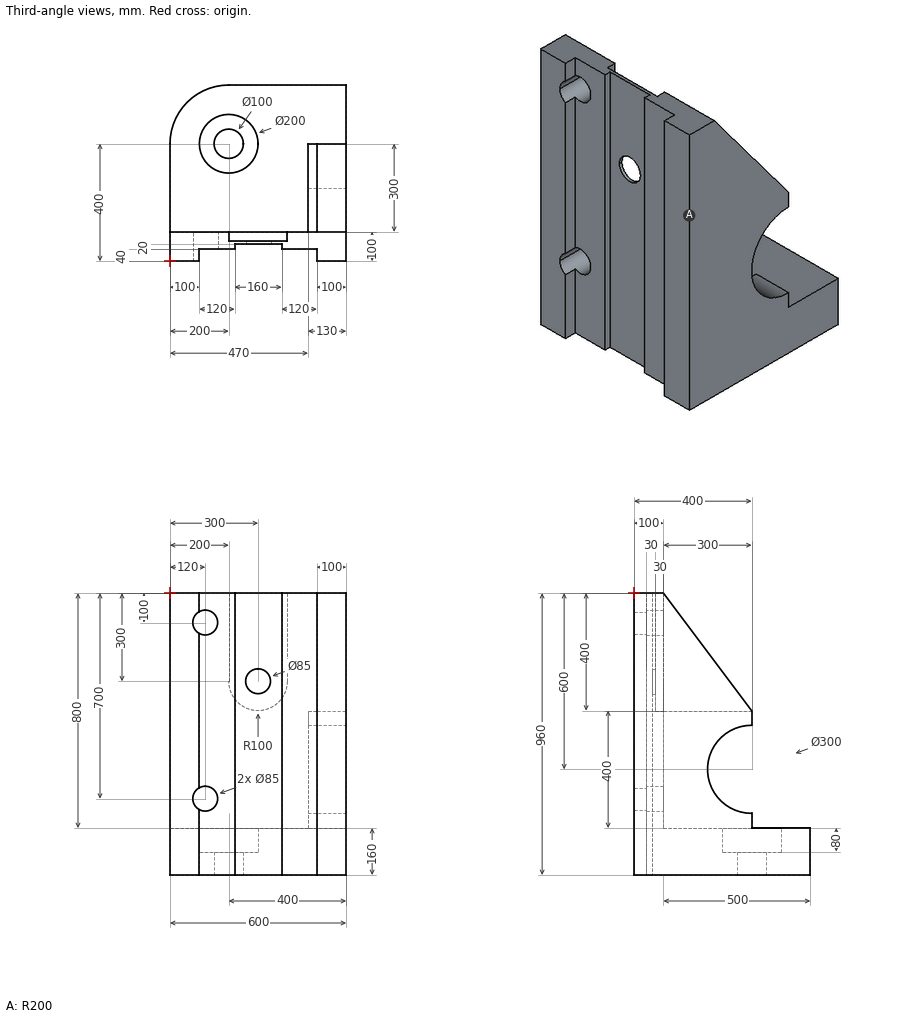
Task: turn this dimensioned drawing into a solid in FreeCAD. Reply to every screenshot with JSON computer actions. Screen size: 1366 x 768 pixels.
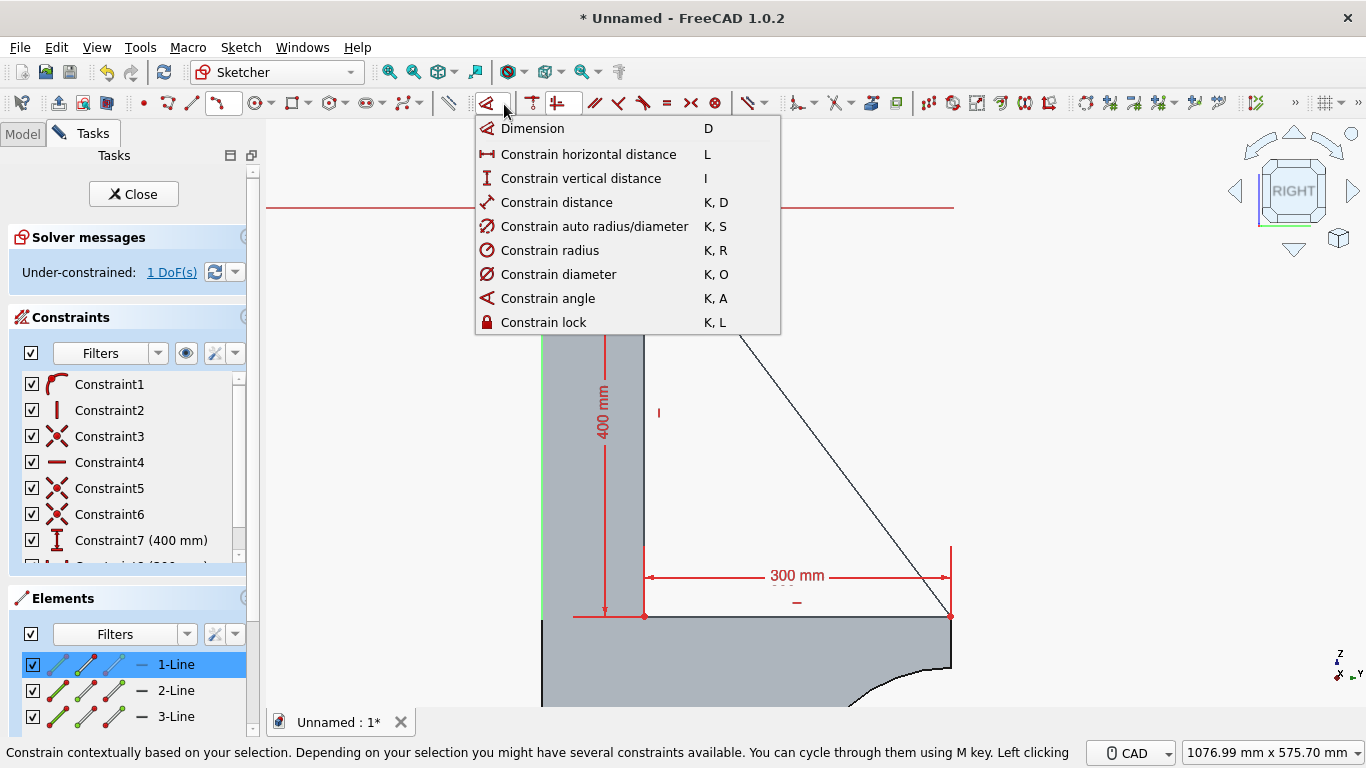
{"action": "left_click", "coordinate": [628, 154]}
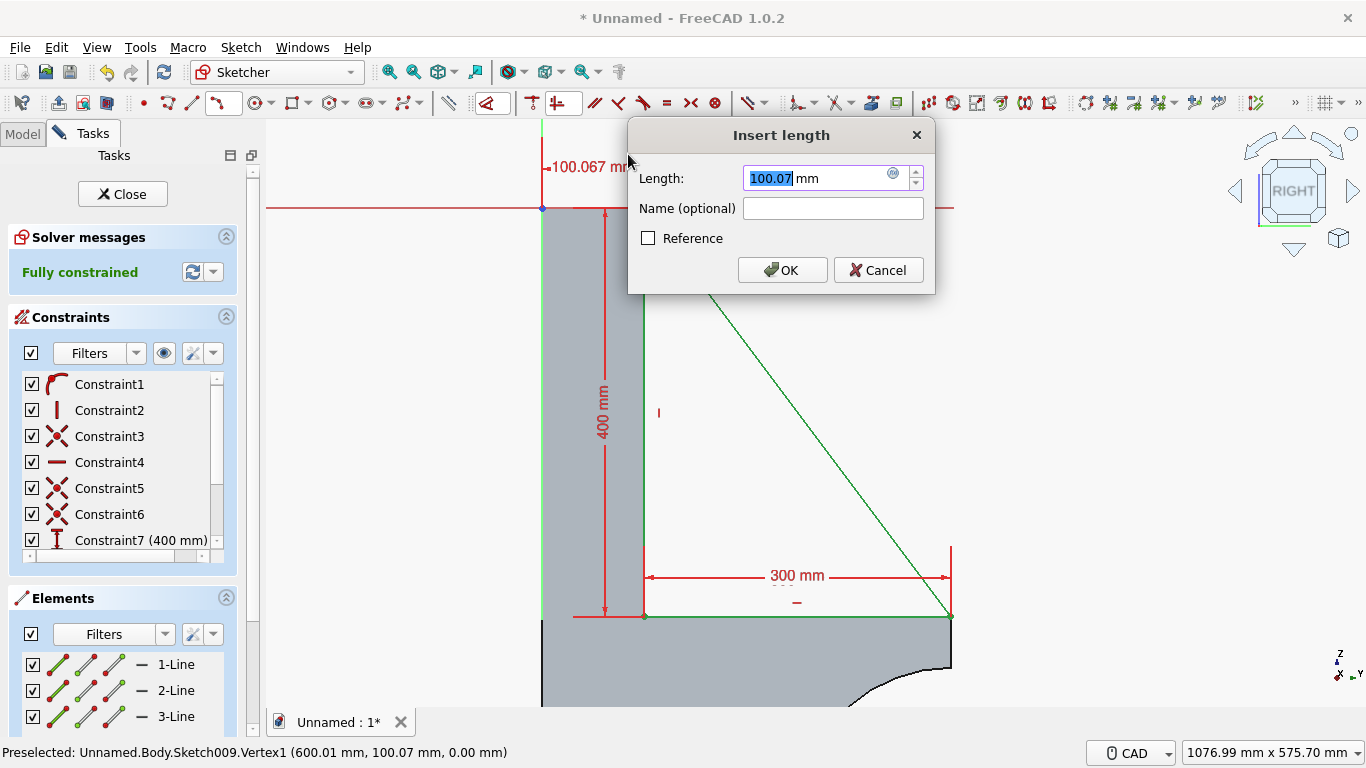
{"action": "type", "text": "100"}
{"action": "key", "text": "Return"}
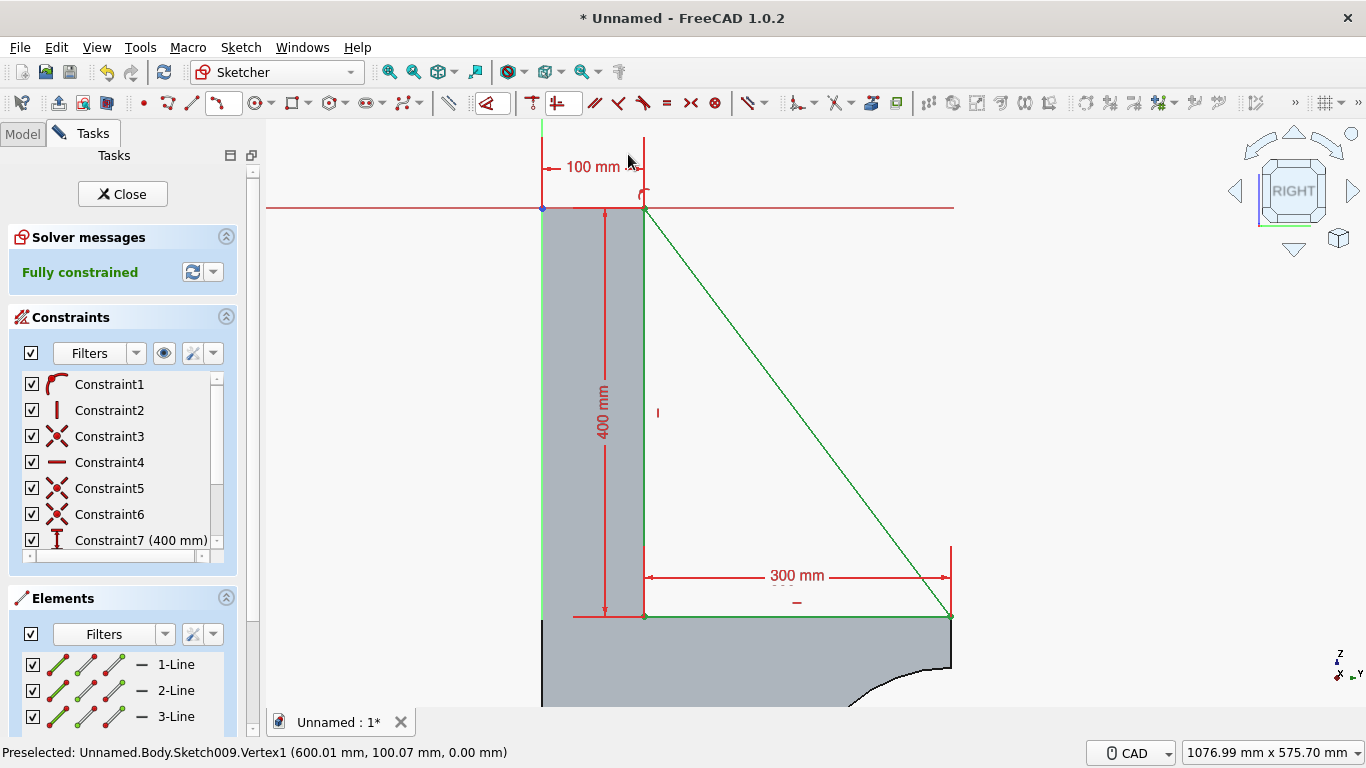
{"action": "left_click", "coordinate": [123, 194]}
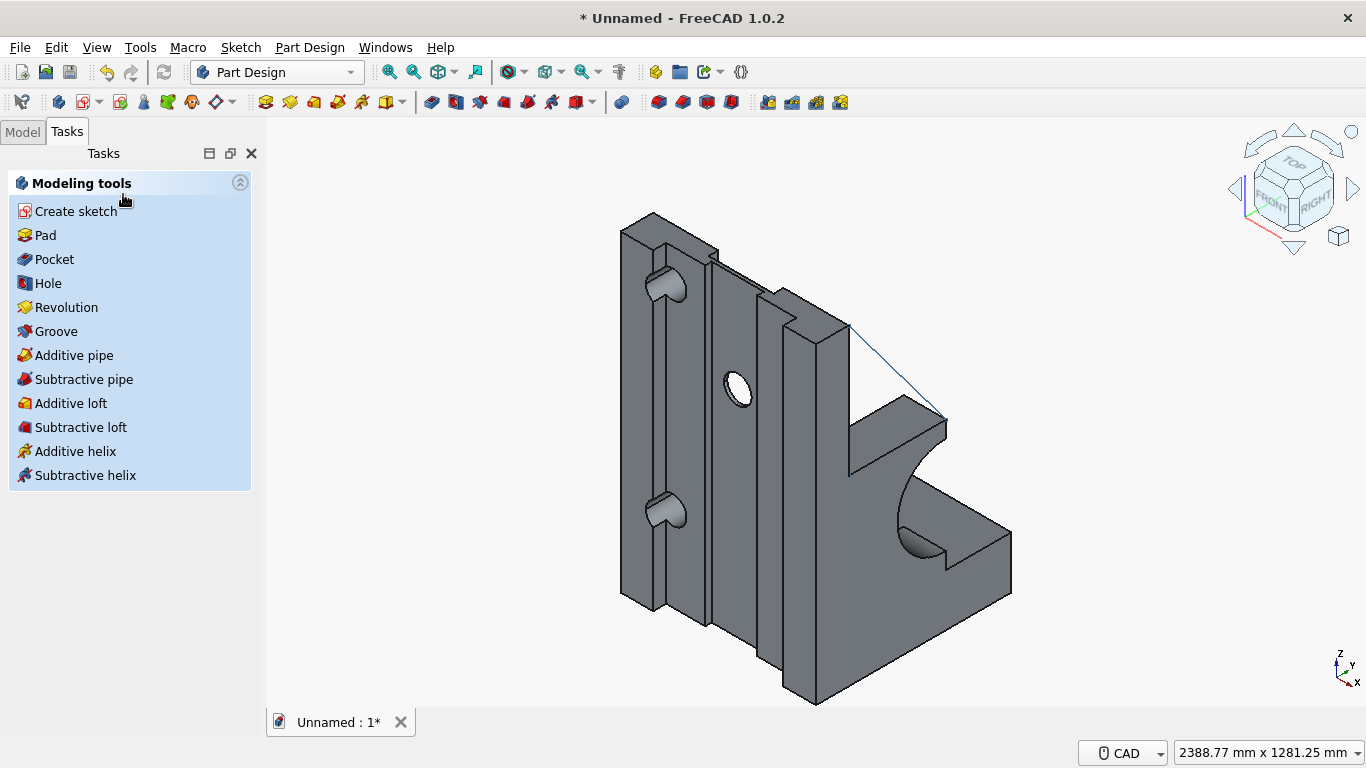
{"action": "left_click", "coordinate": [266, 102]}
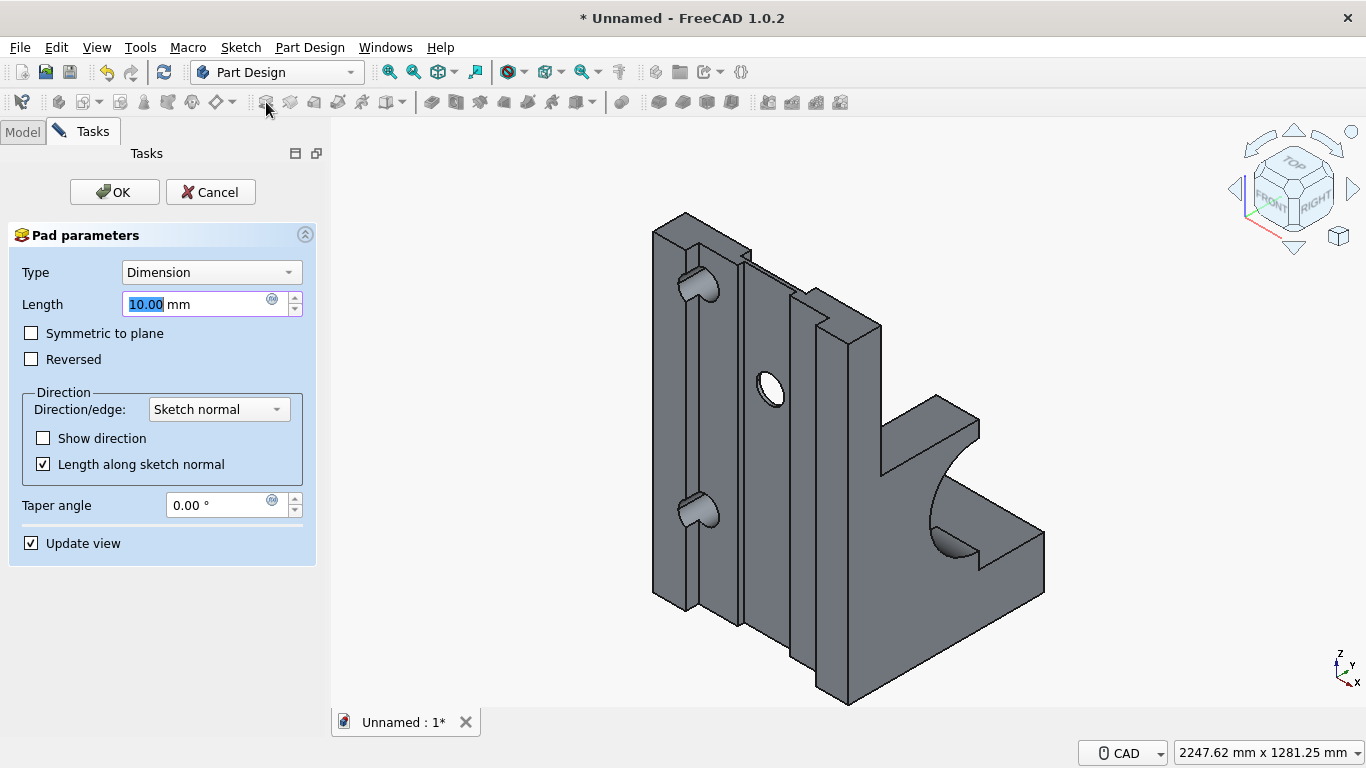
{"action": "type", "text": "100"}
{"action": "key", "text": "Tab"}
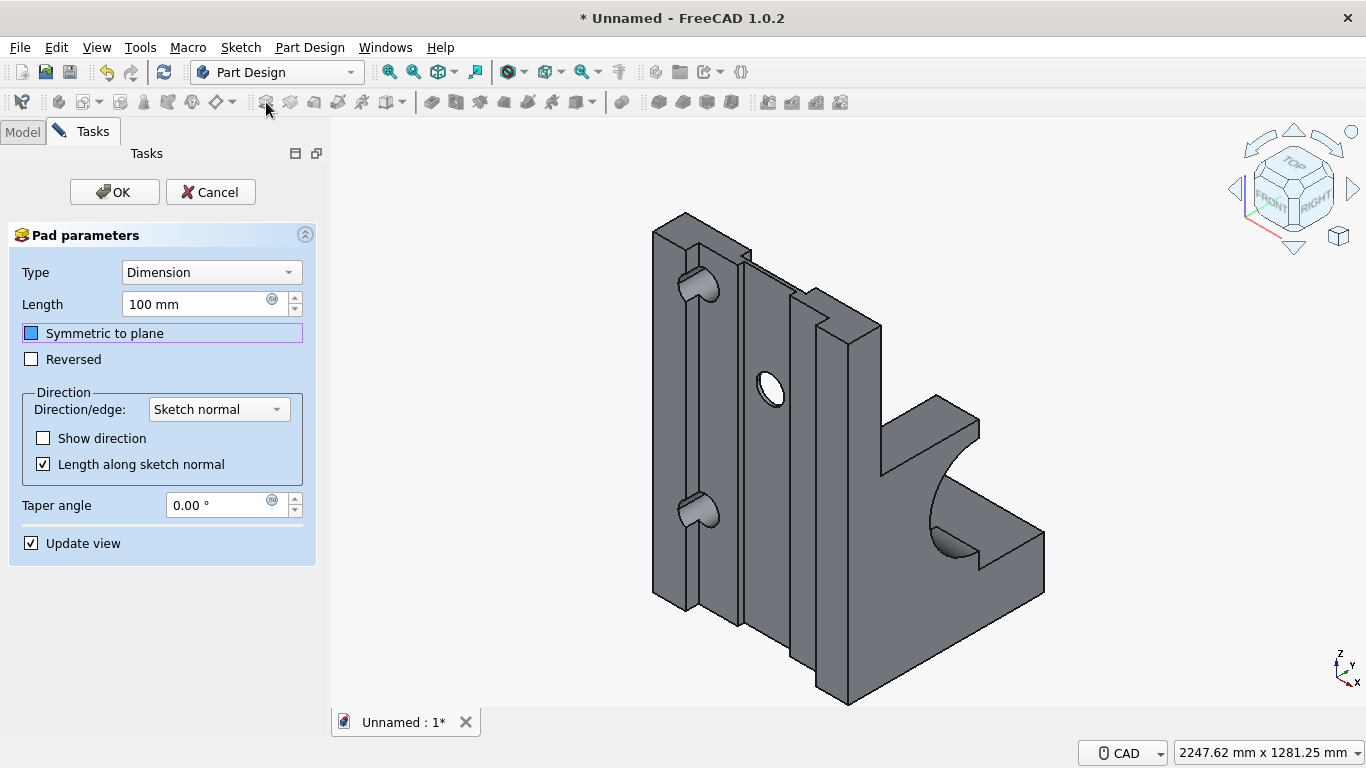
{"action": "left_click", "coordinate": [30, 359]}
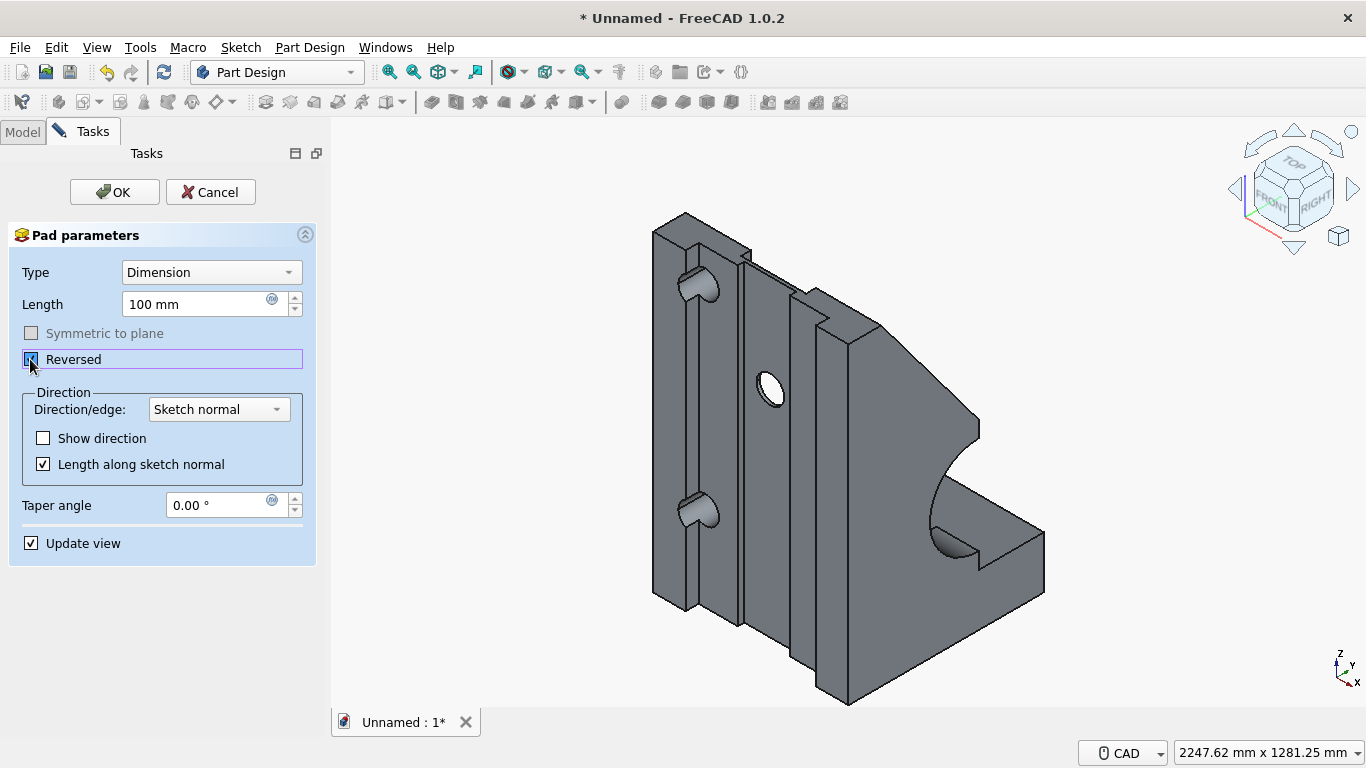
{"action": "left_click", "coordinate": [115, 192]}